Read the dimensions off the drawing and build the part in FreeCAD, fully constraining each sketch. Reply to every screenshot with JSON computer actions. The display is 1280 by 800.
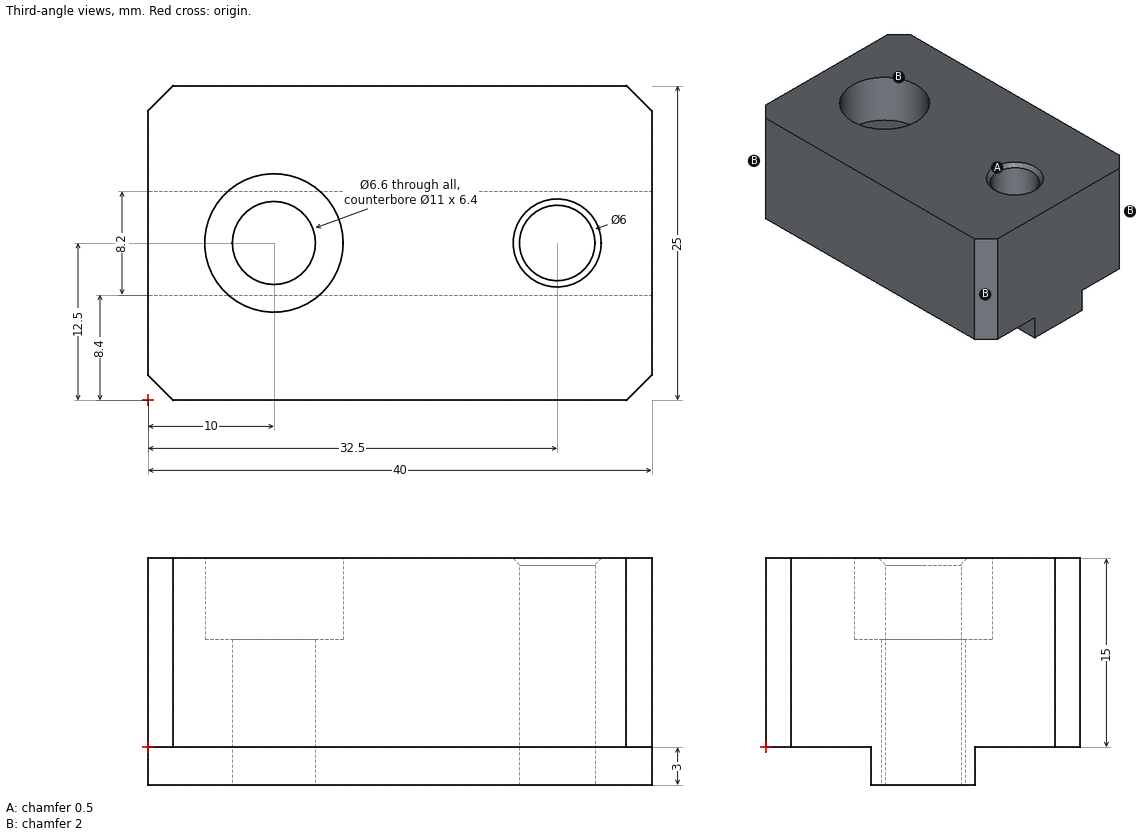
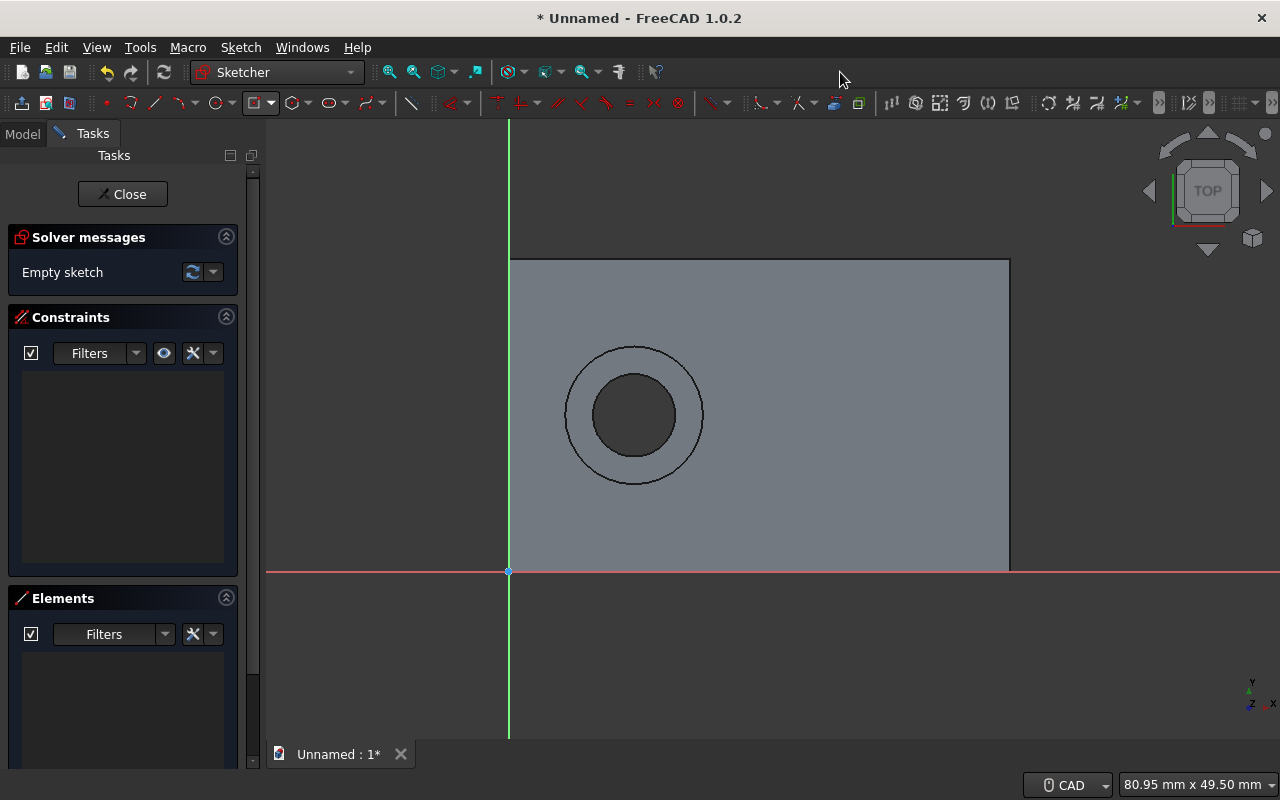
{"action": "scroll", "coordinate": [969, 412], "scroll_direction": "up", "scroll_amount": 8}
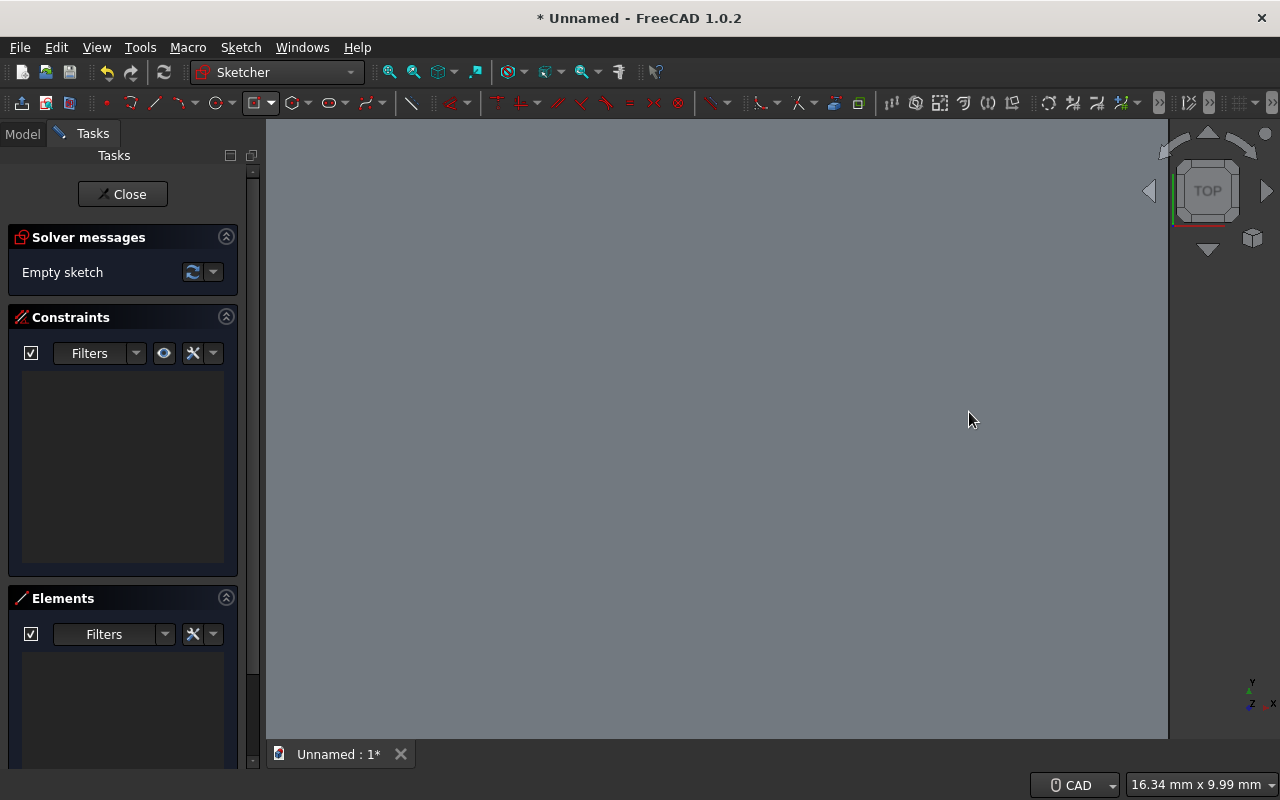
{"action": "left_click", "coordinate": [216, 104]}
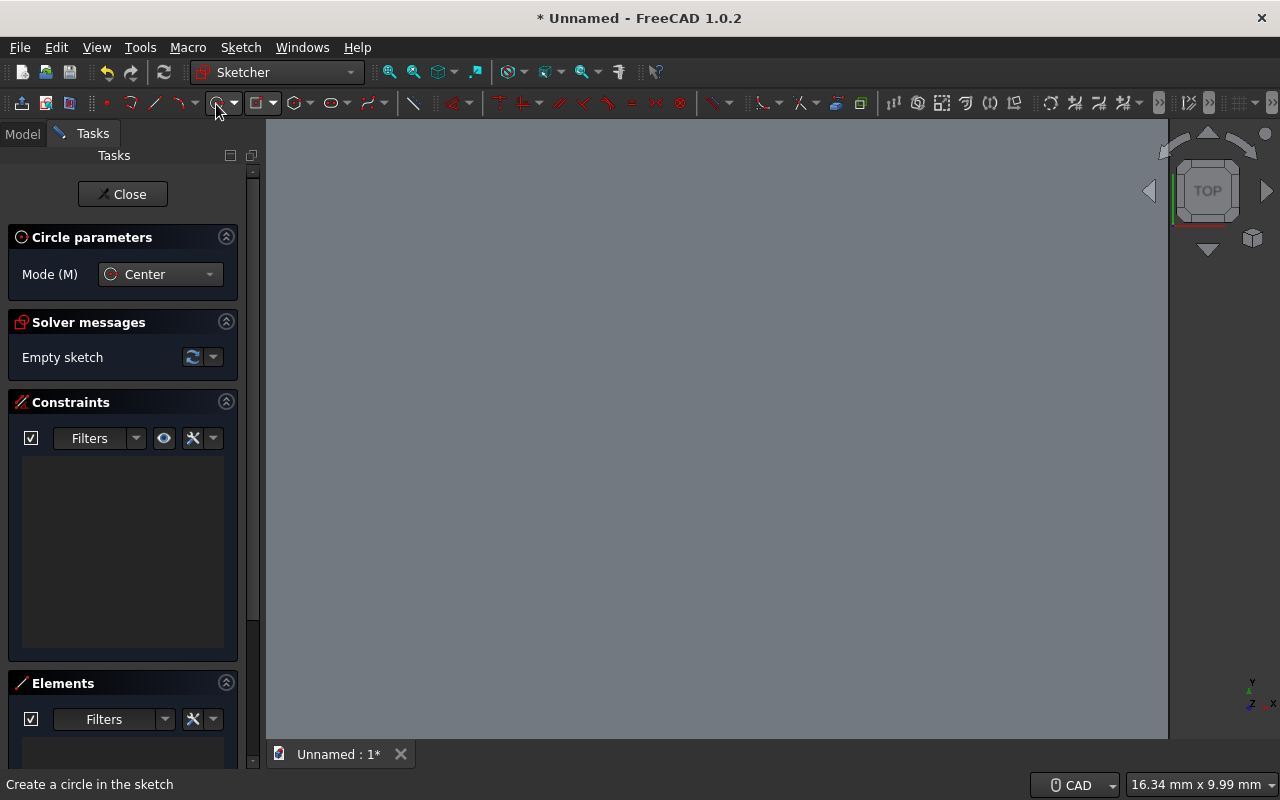
{"action": "left_click", "coordinate": [703, 427]}
{"action": "left_click", "coordinate": [835, 295]}
{"action": "key", "text": "Escape"}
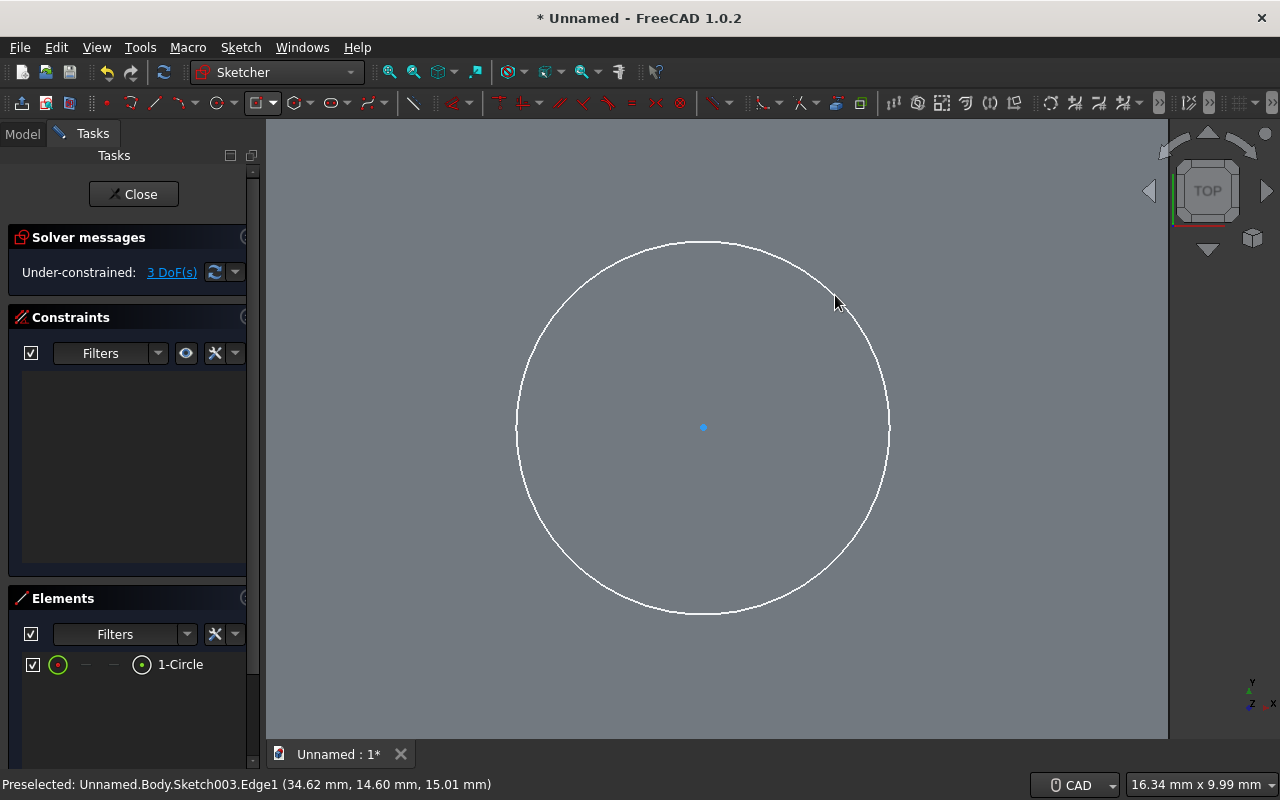
{"action": "left_click", "coordinate": [452, 104]}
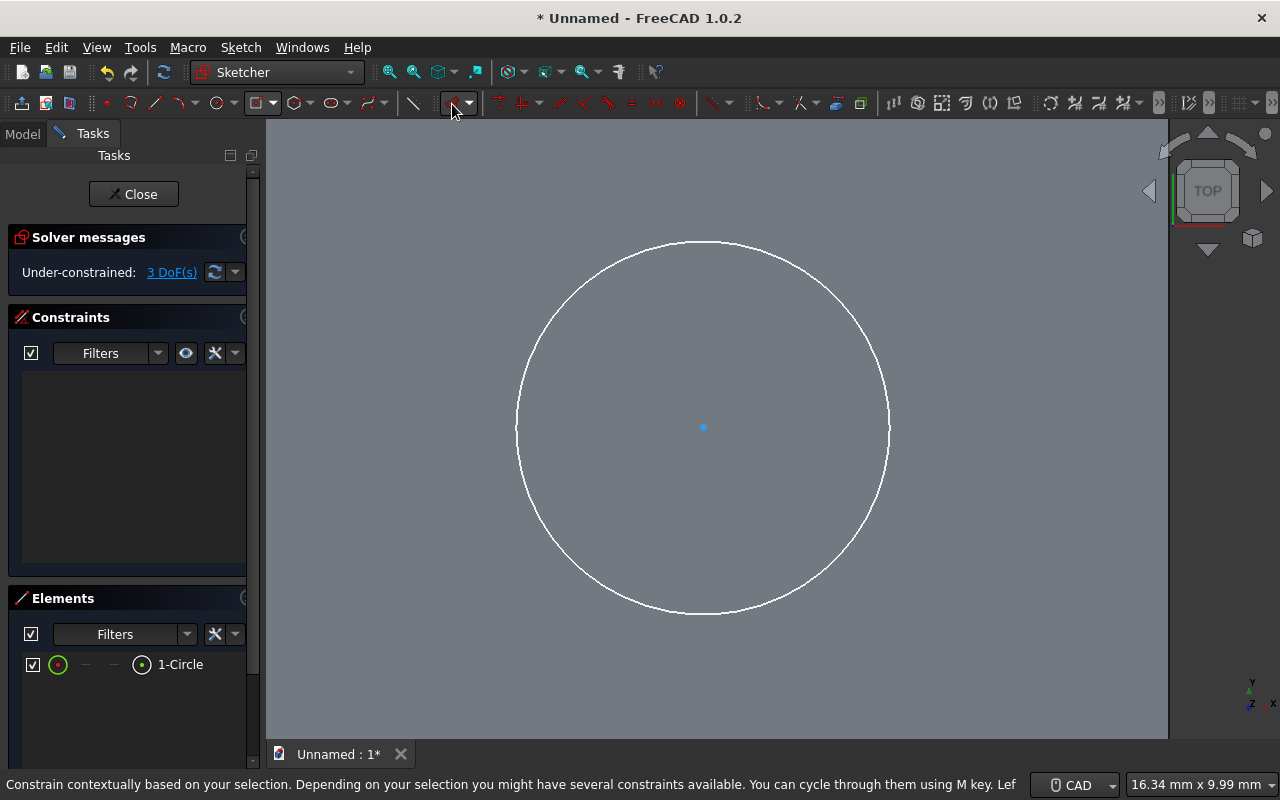
{"action": "left_click", "coordinate": [835, 296]}
{"action": "left_click", "coordinate": [858, 273]}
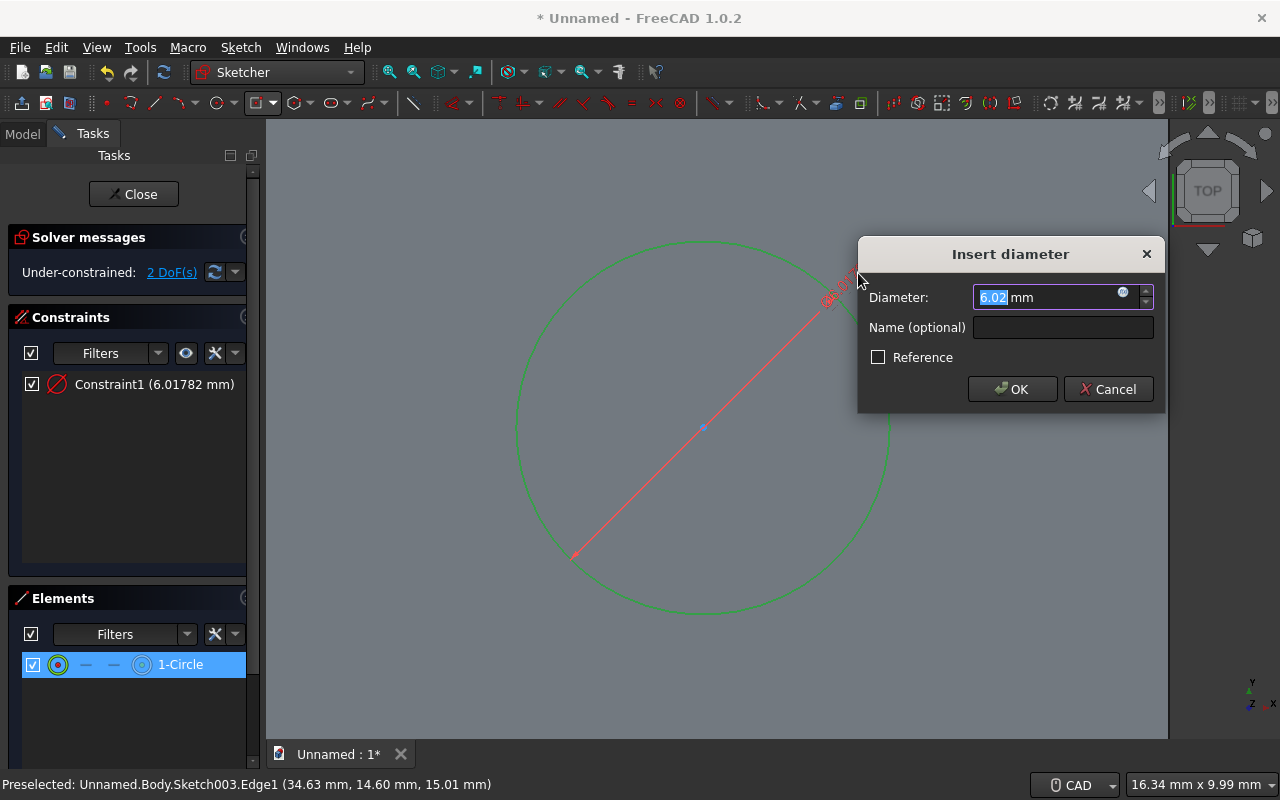
{"action": "type", "text": "6"}
{"action": "key", "text": "Return"}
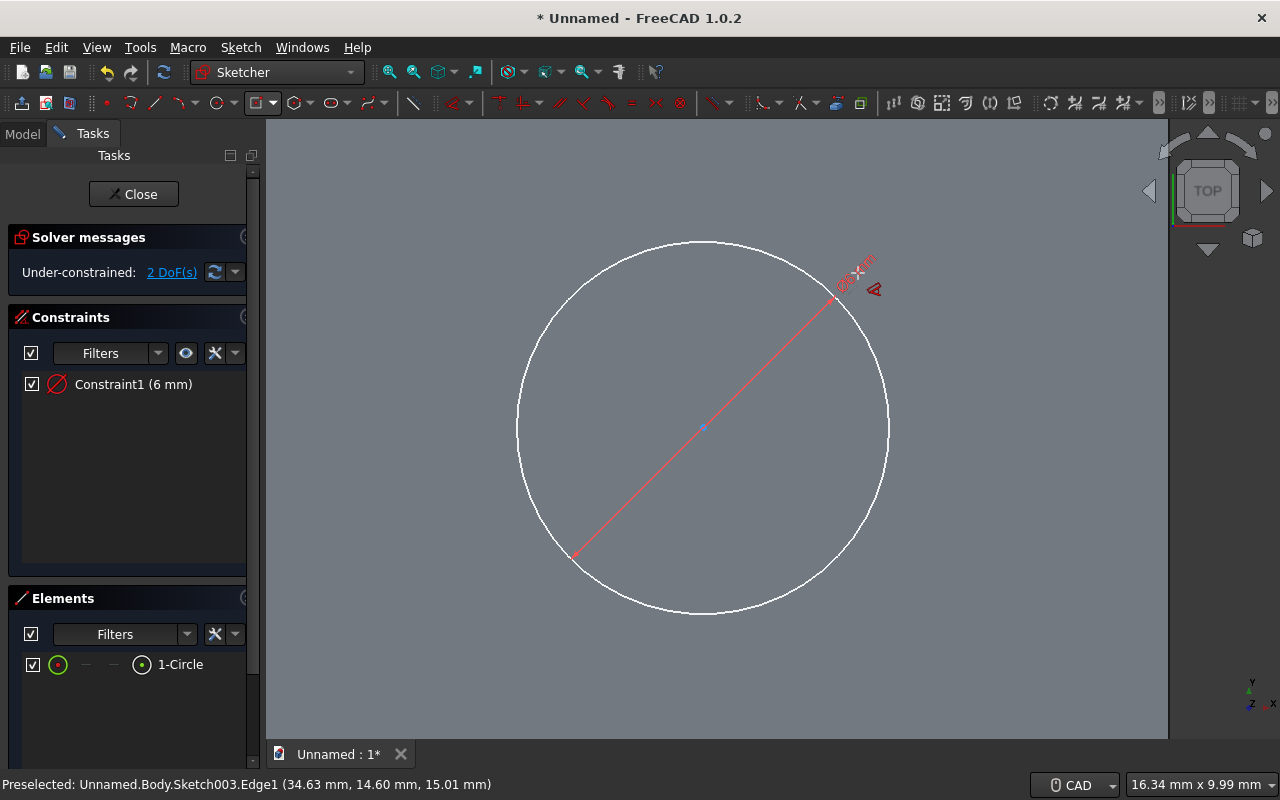
{"action": "left_click", "coordinate": [703, 428]}
{"action": "left_click", "coordinate": [498, 394]}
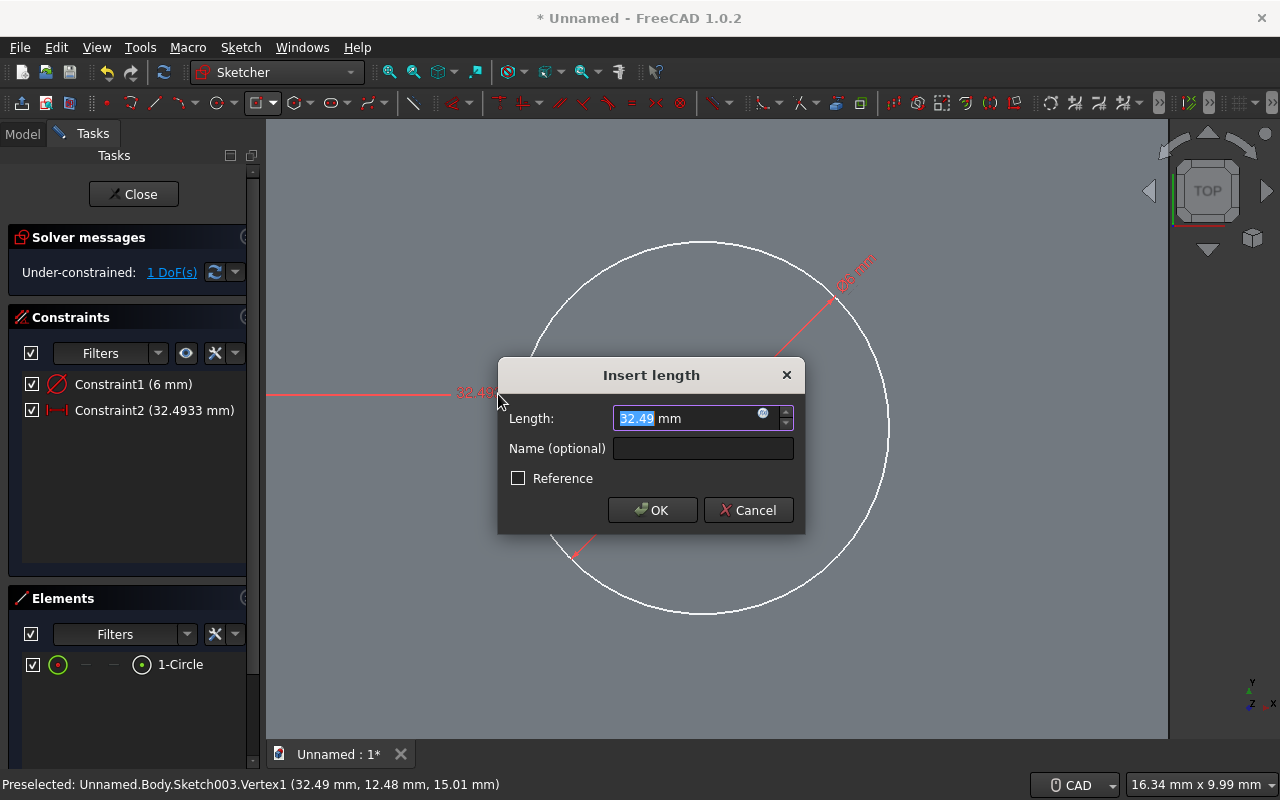
{"action": "type", "text": "32.5"}
{"action": "key", "text": "Return"}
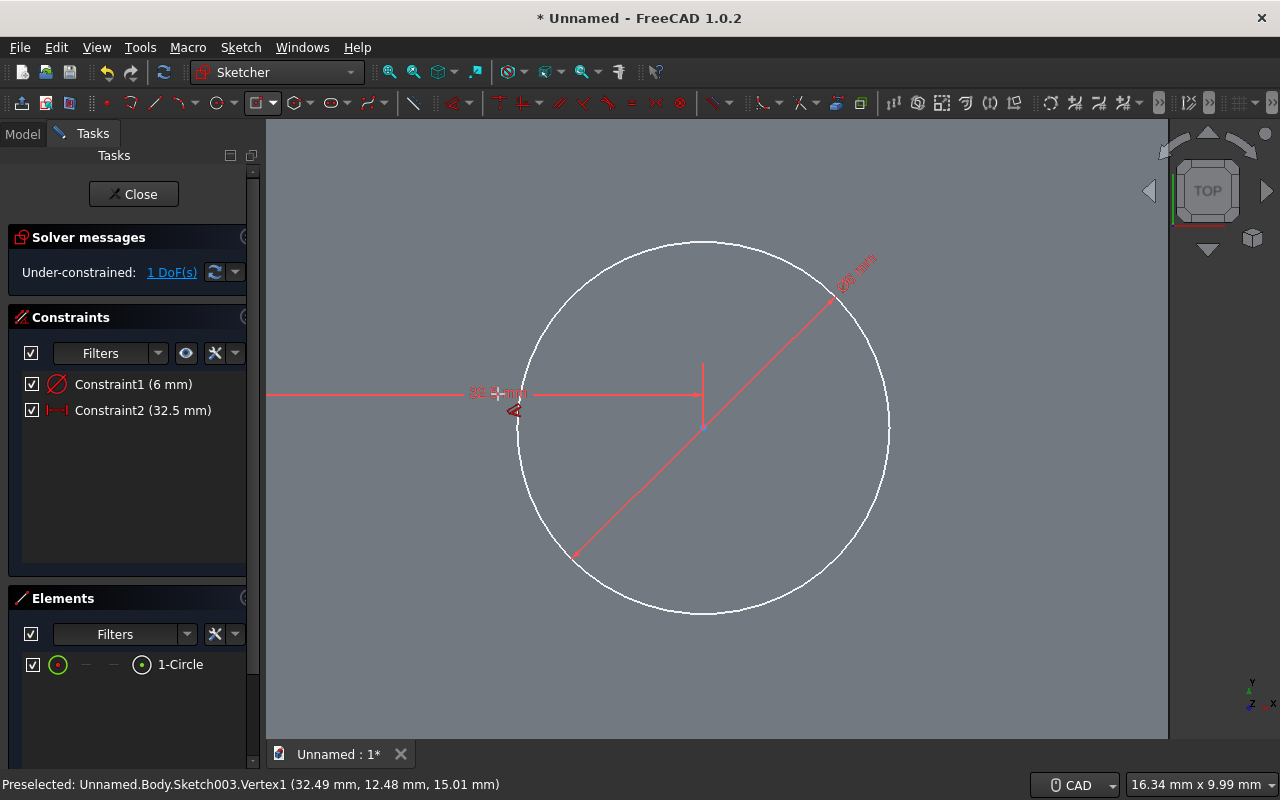
{"action": "left_click", "coordinate": [703, 428]}
{"action": "left_click", "coordinate": [737, 570]}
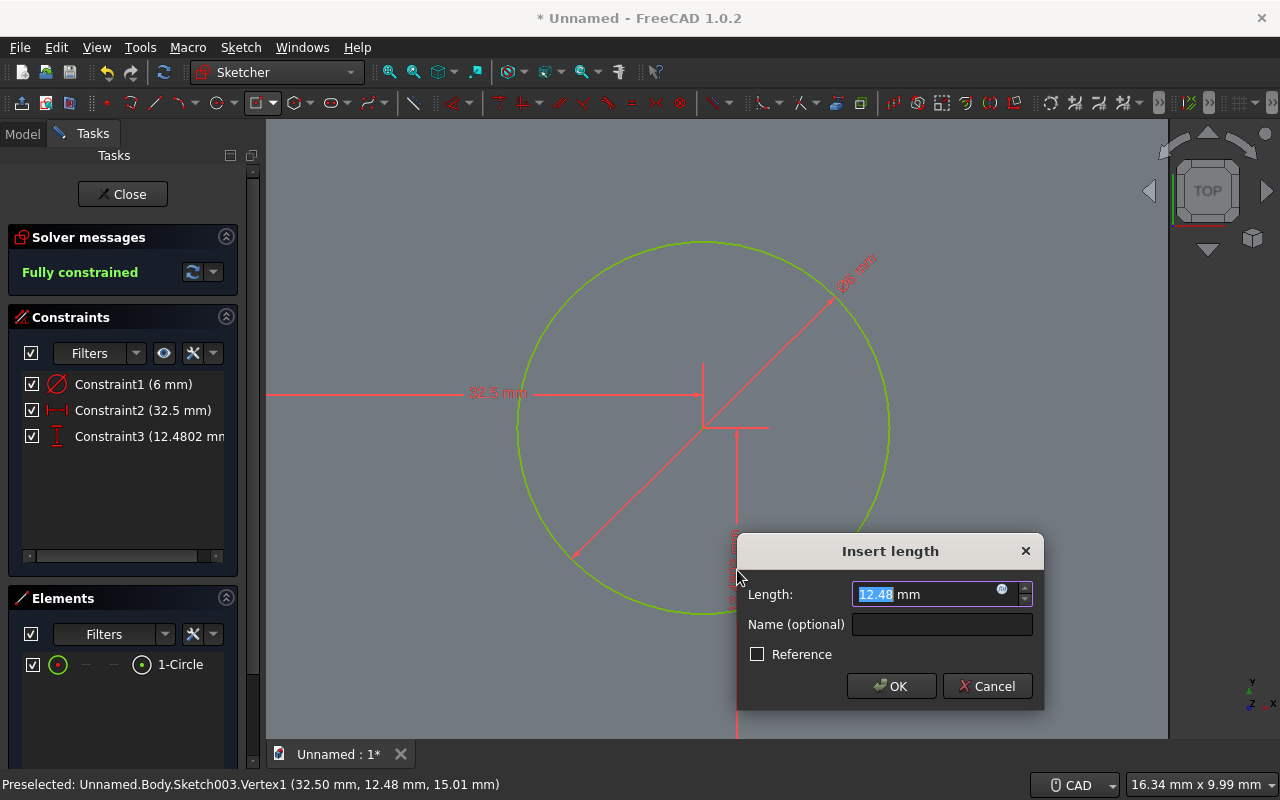
{"action": "type", "text": "12.5"}
{"action": "key", "text": "Return"}
{"action": "key", "text": "Escape"}